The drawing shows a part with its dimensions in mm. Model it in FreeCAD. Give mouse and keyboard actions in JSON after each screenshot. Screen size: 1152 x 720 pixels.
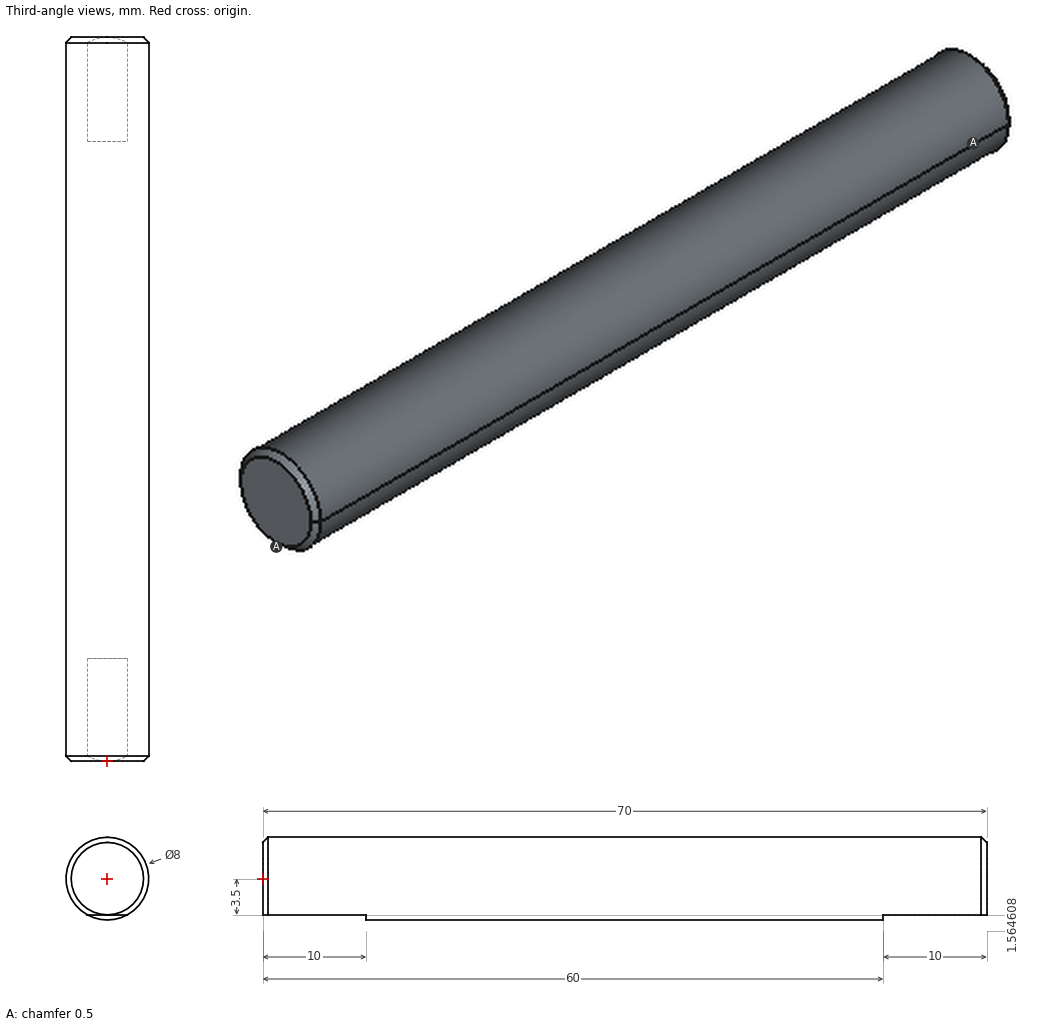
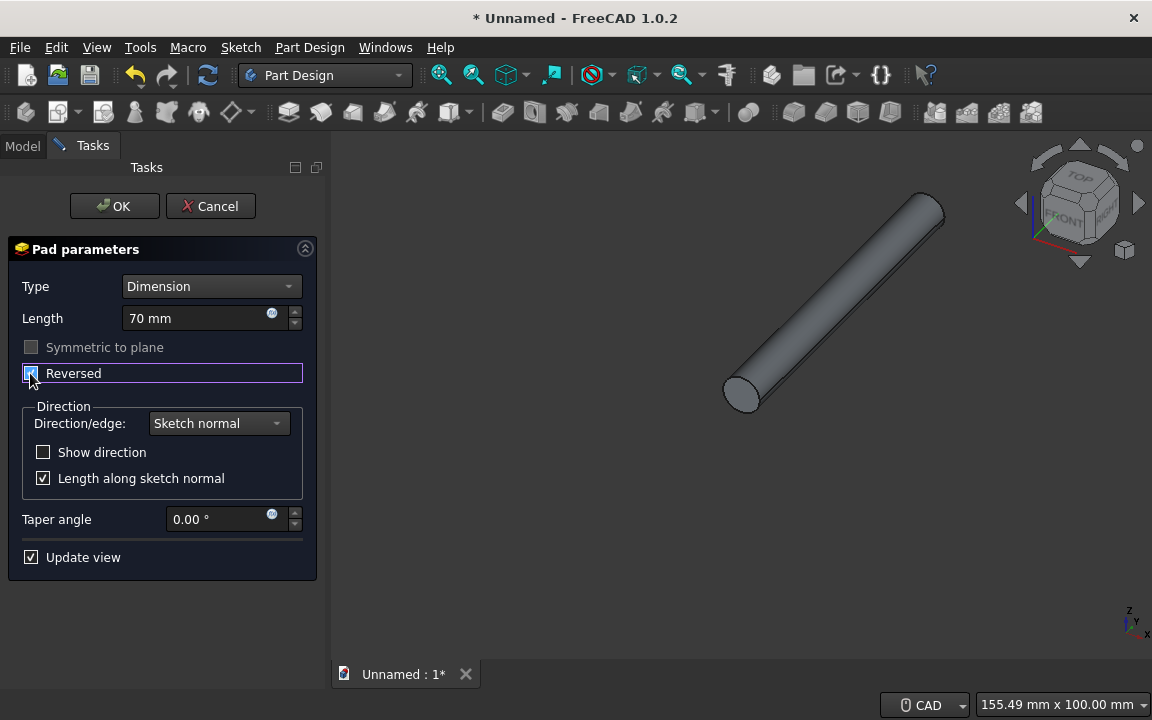
{"action": "left_click", "coordinate": [115, 206]}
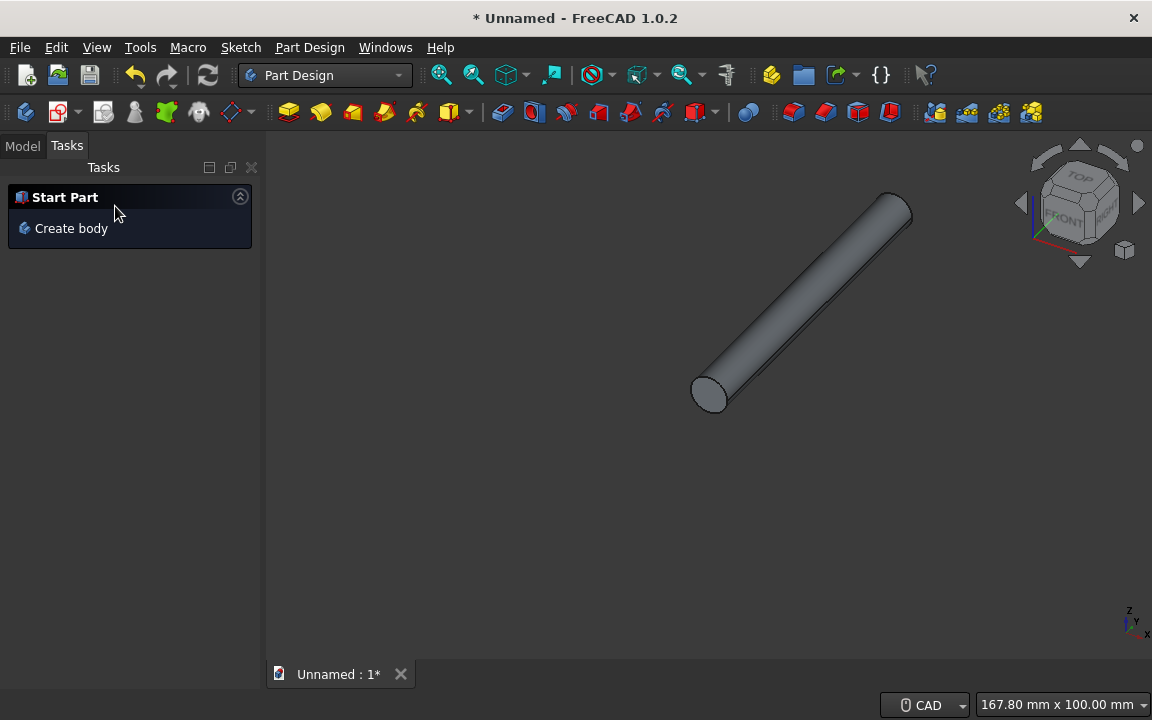
{"action": "key", "text": "v f"}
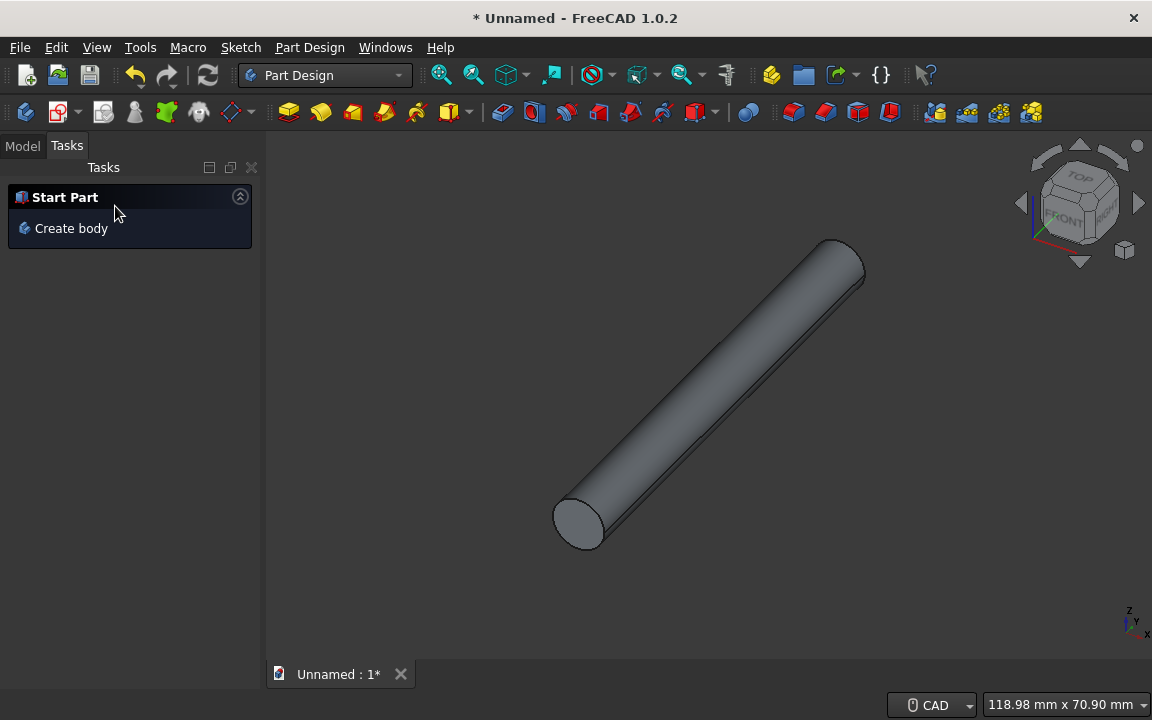
{"action": "left_click", "coordinate": [558, 502]}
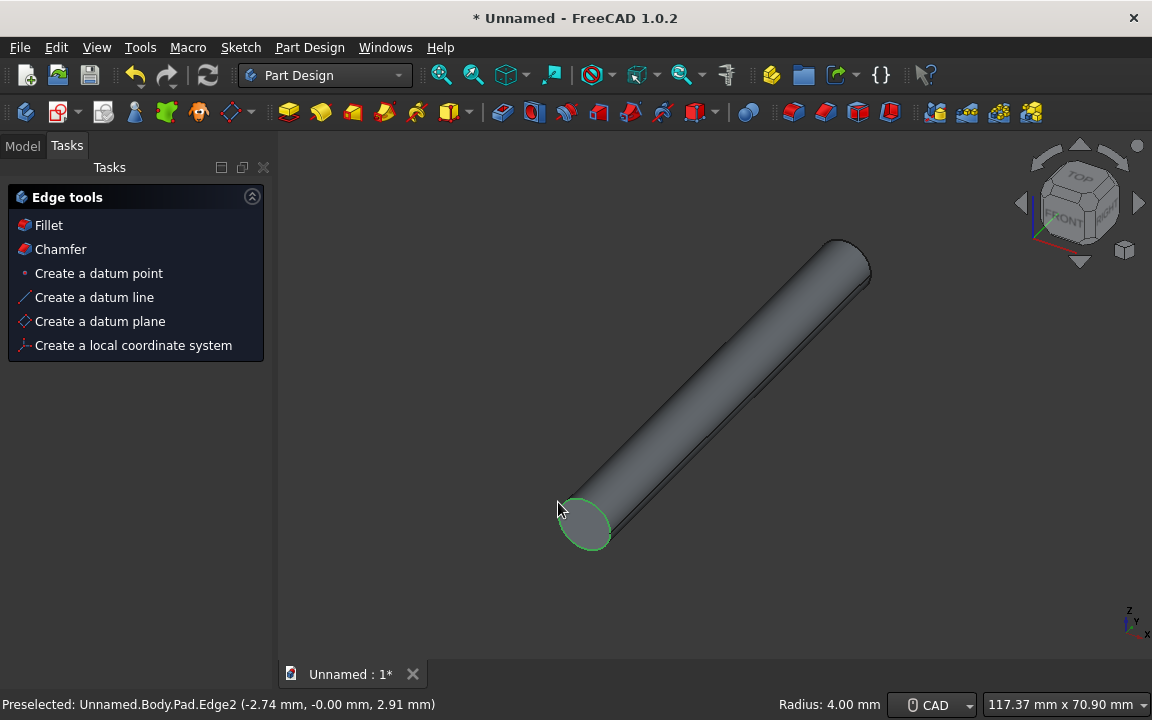
{"action": "key", "text": "0"}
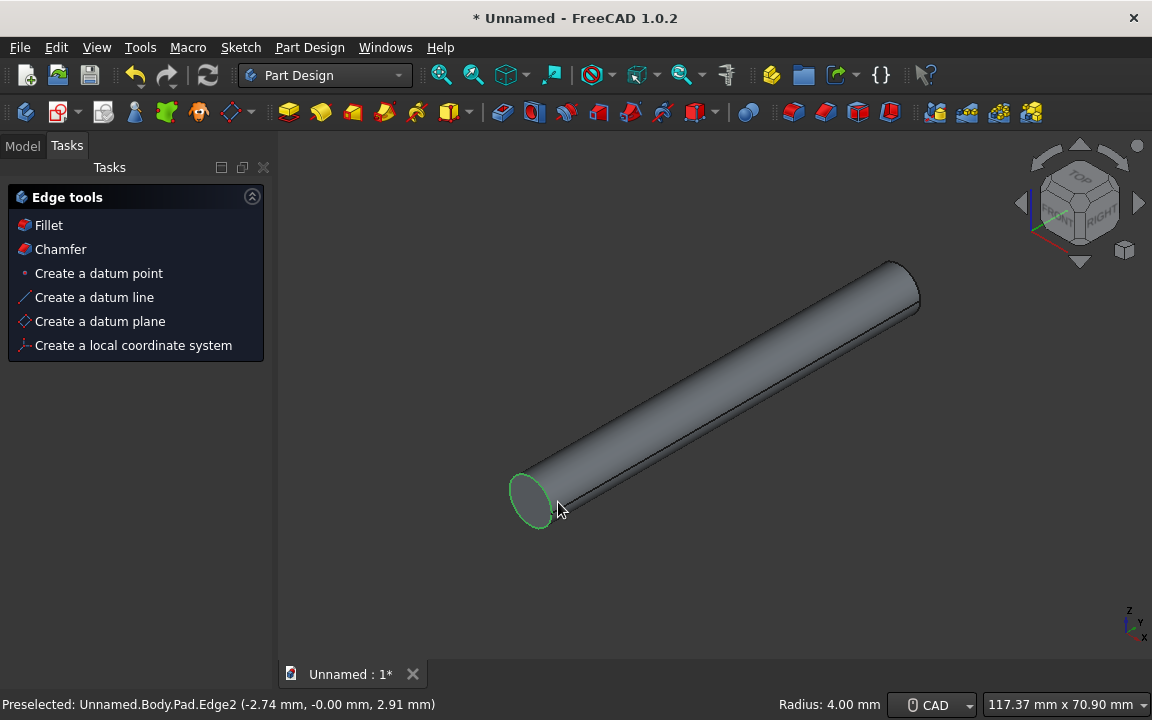
{"action": "left_click", "coordinate": [906, 268], "text": "ctrl"}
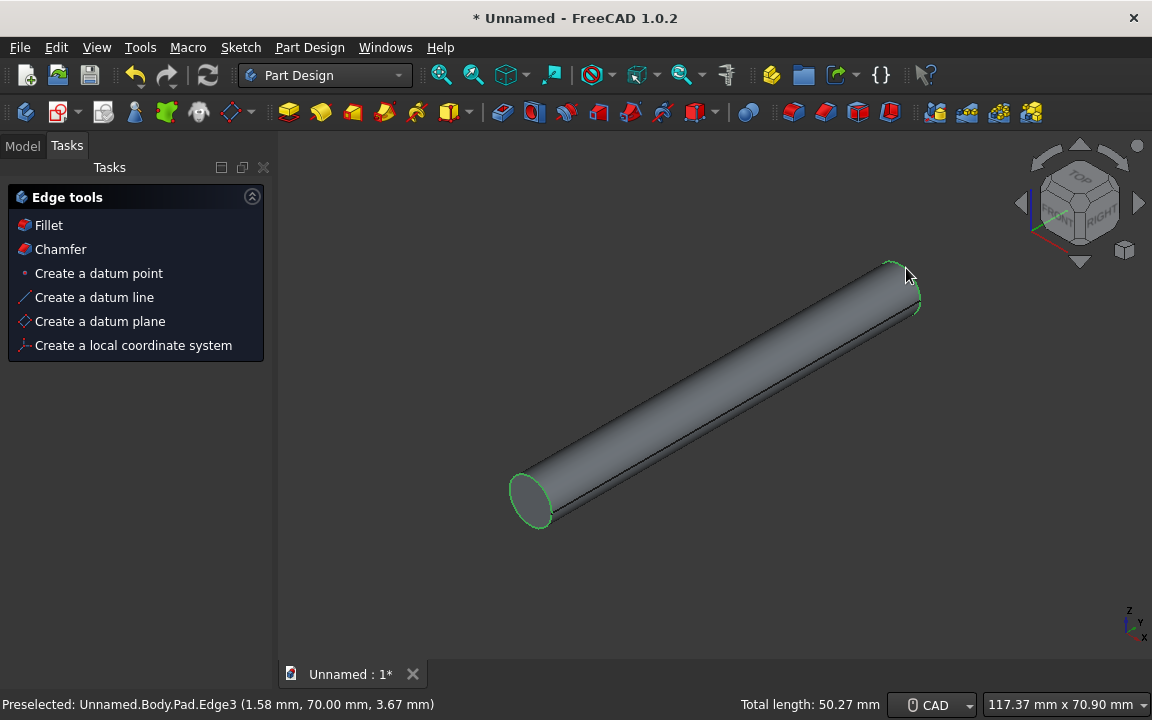
{"action": "left_click", "coordinate": [826, 112]}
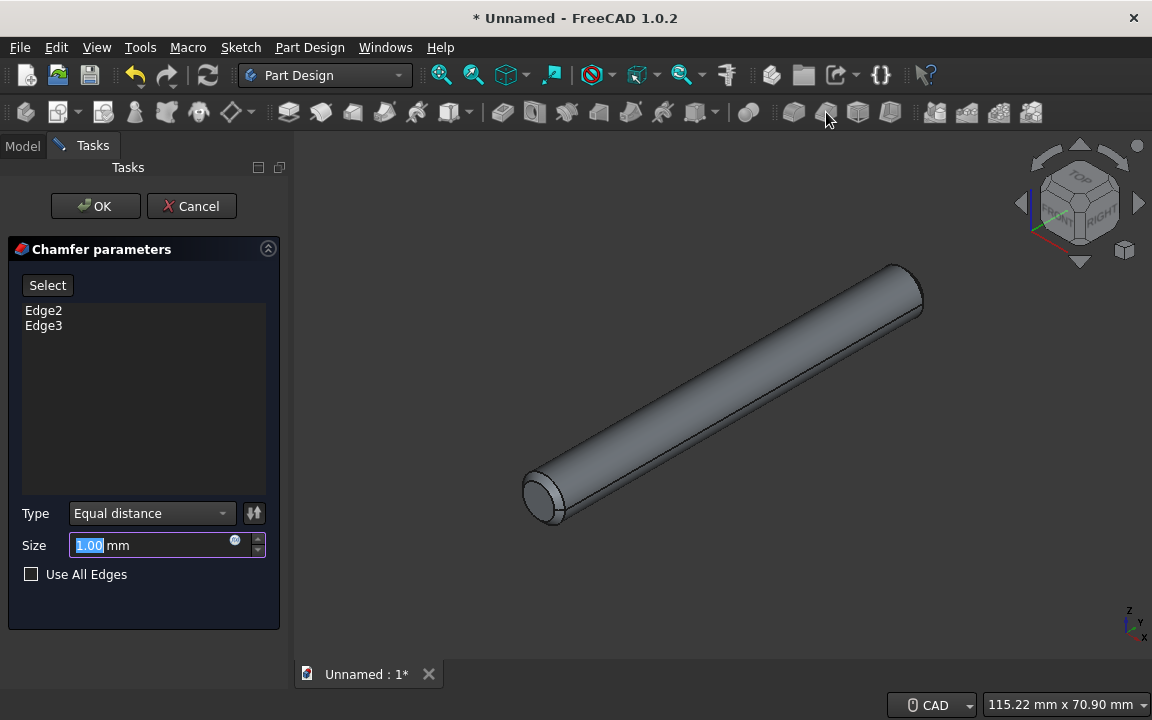
{"action": "type", "text": "0.5"}
{"action": "key", "text": "Tab"}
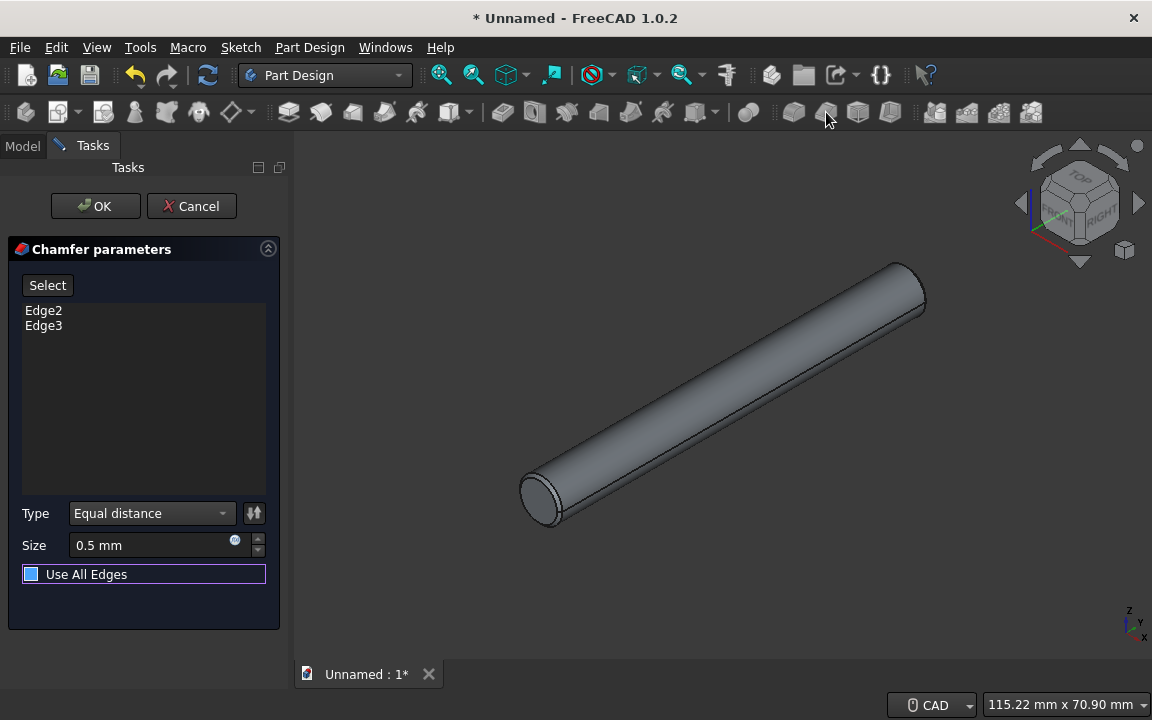
{"action": "left_click", "coordinate": [96, 206]}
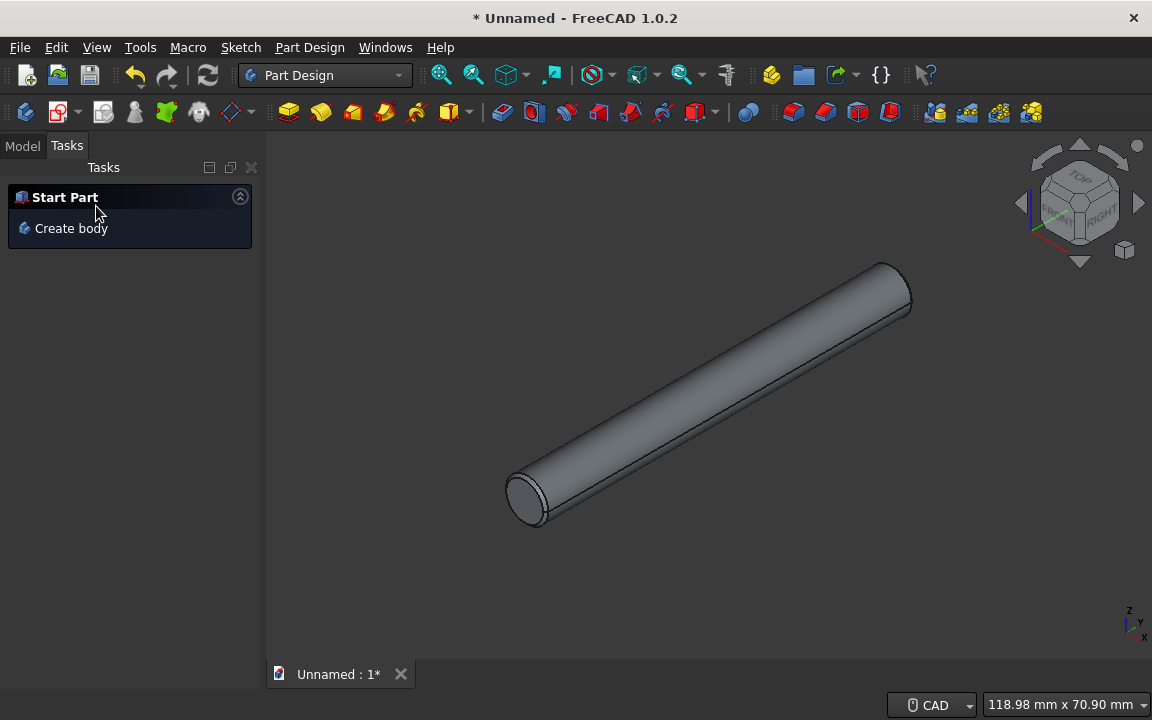
{"action": "left_click", "coordinate": [58, 112]}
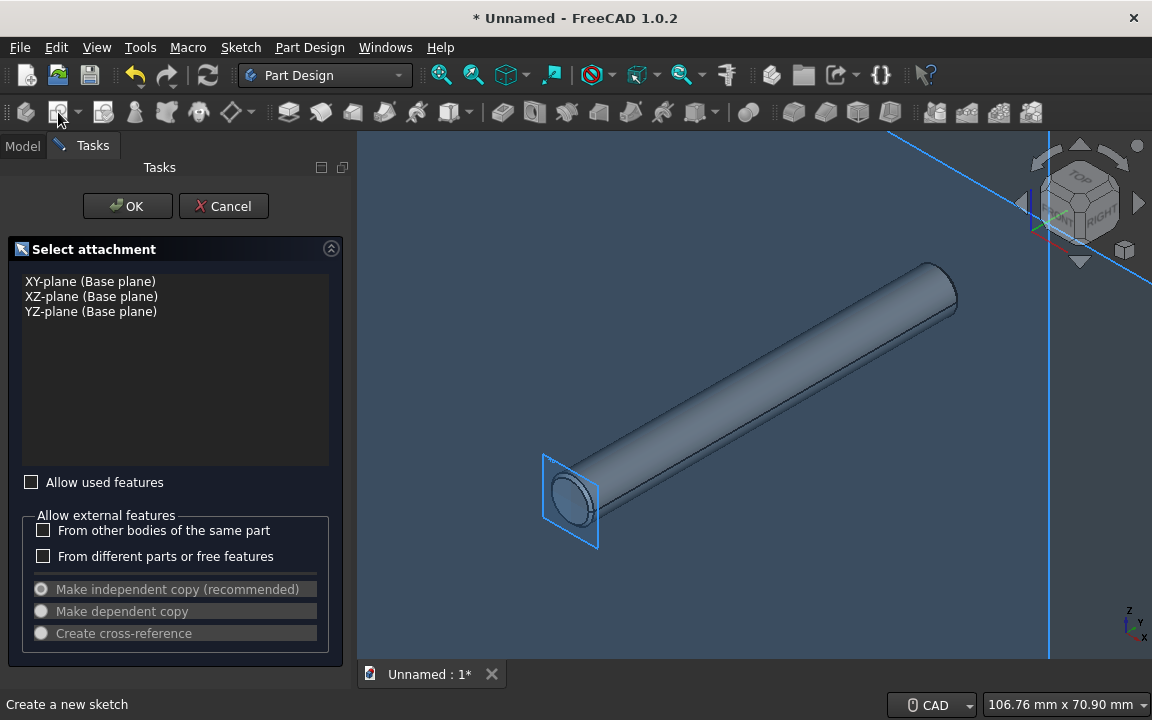
{"action": "left_click", "coordinate": [82, 312]}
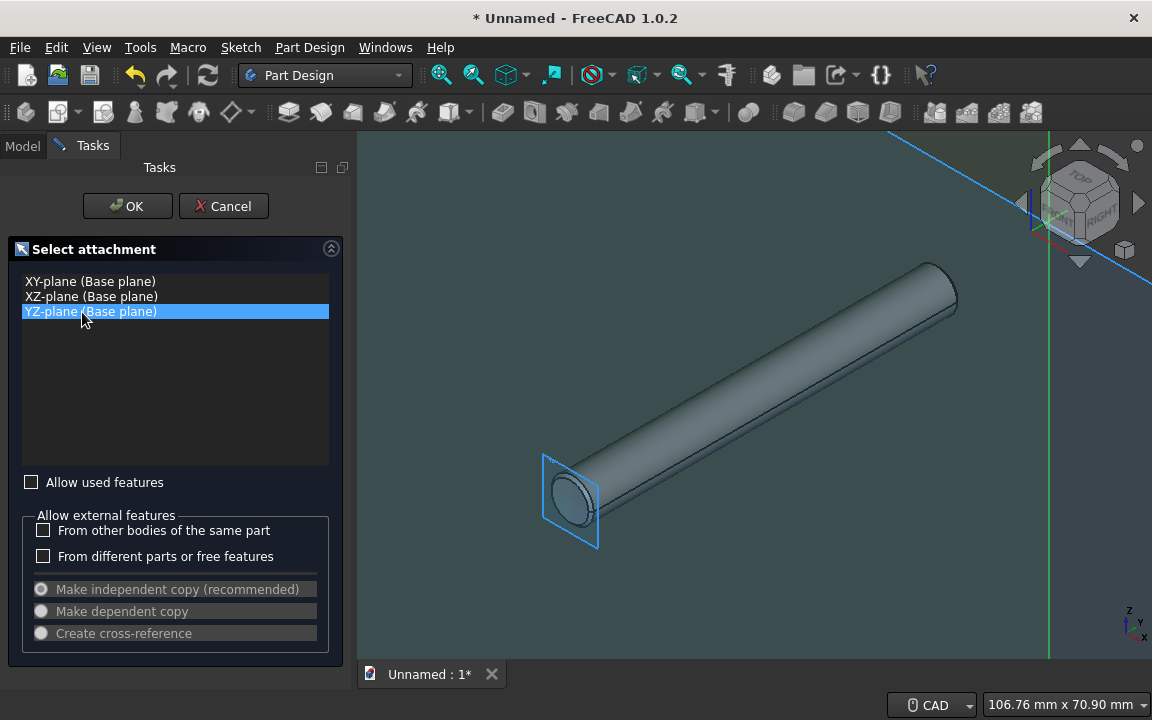
{"action": "left_click", "coordinate": [128, 206]}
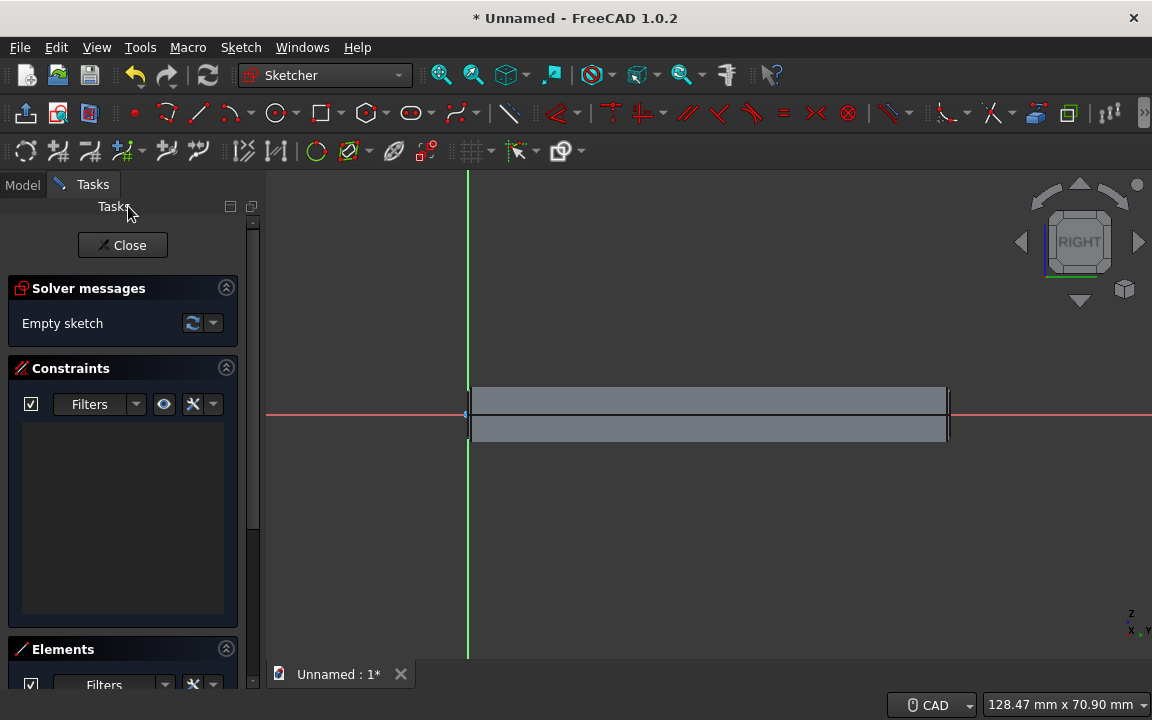
{"action": "left_click", "coordinate": [90, 114]}